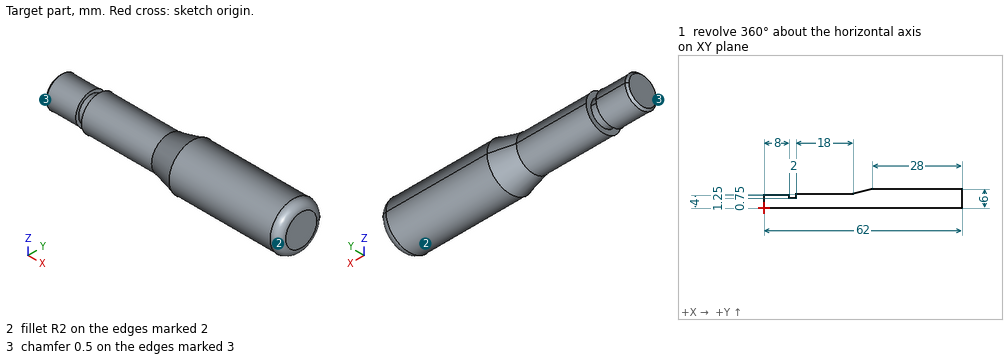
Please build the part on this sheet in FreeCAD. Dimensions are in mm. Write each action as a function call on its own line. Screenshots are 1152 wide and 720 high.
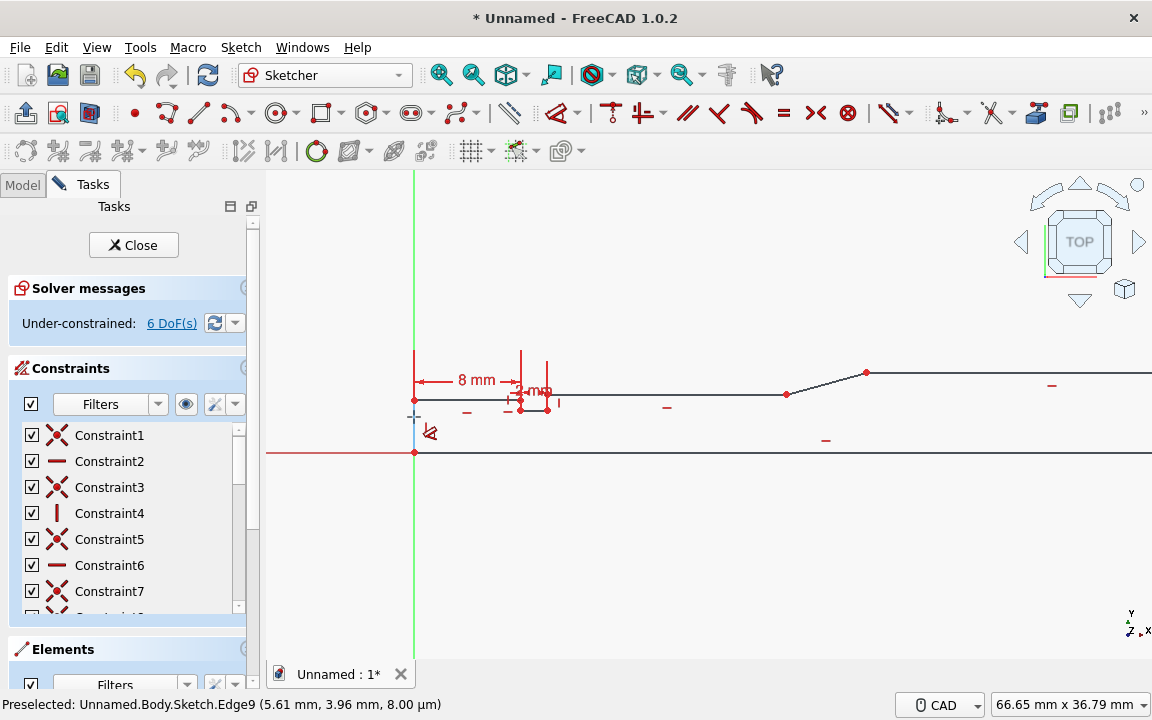
click(414, 416)
click(380, 426)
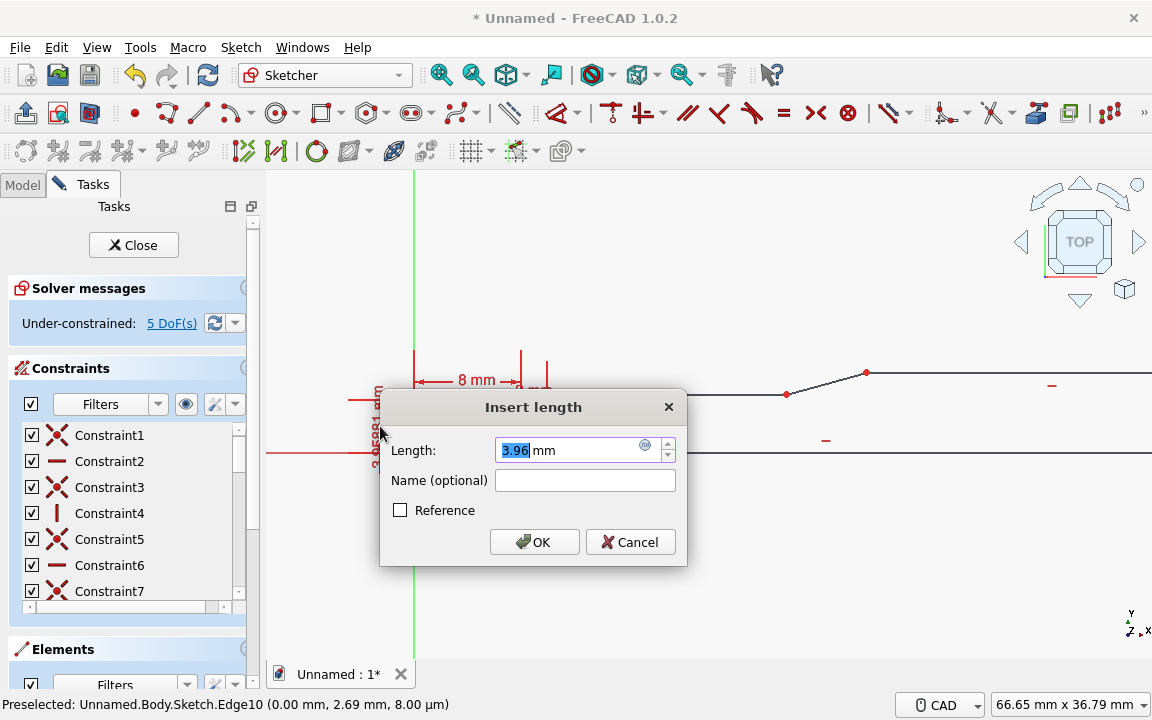
text(4)
key(Return)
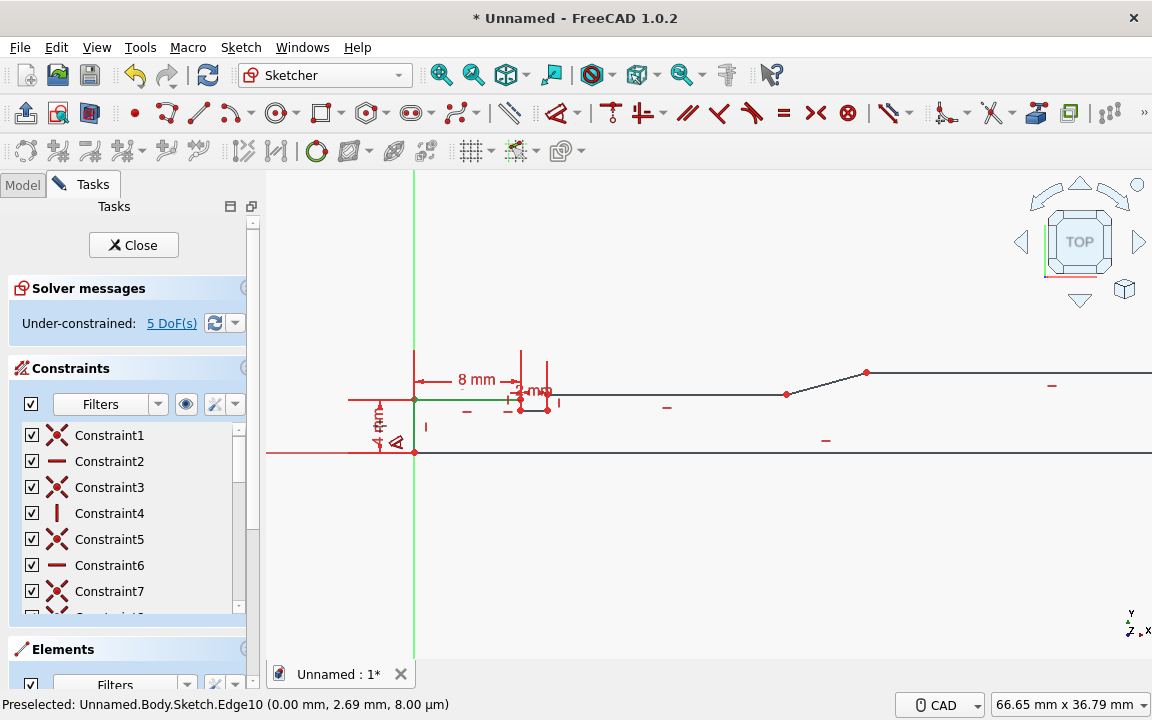
click(662, 453)
click(701, 487)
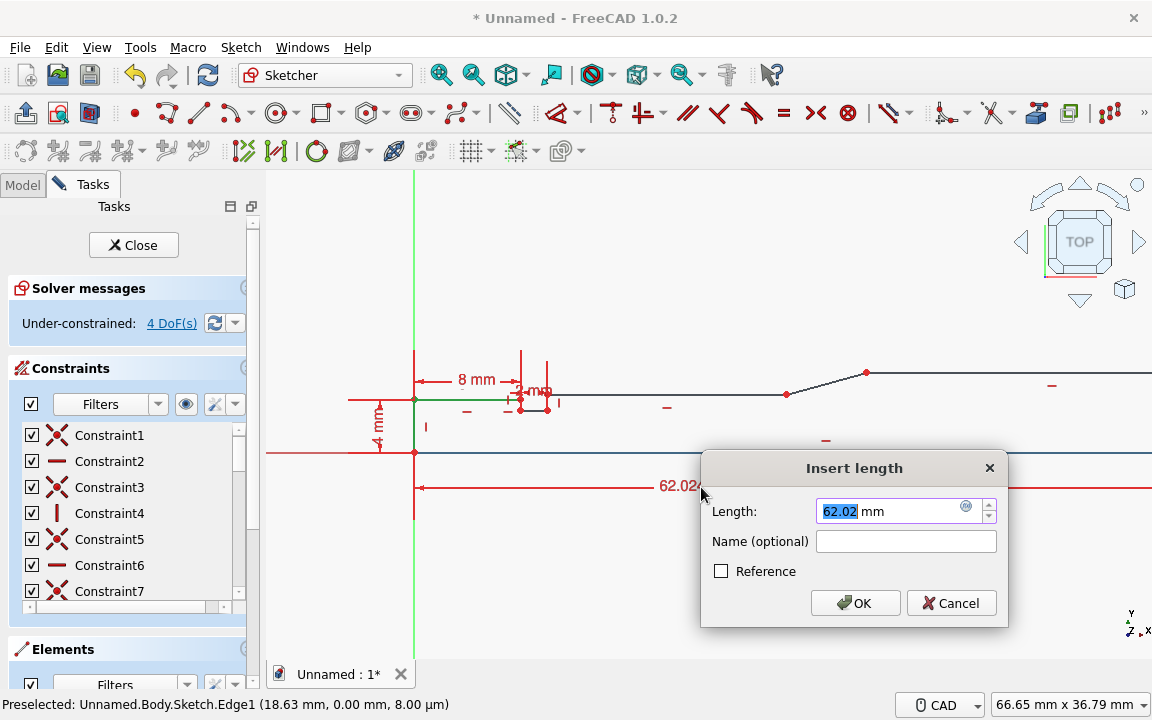
text(62)
key(Return)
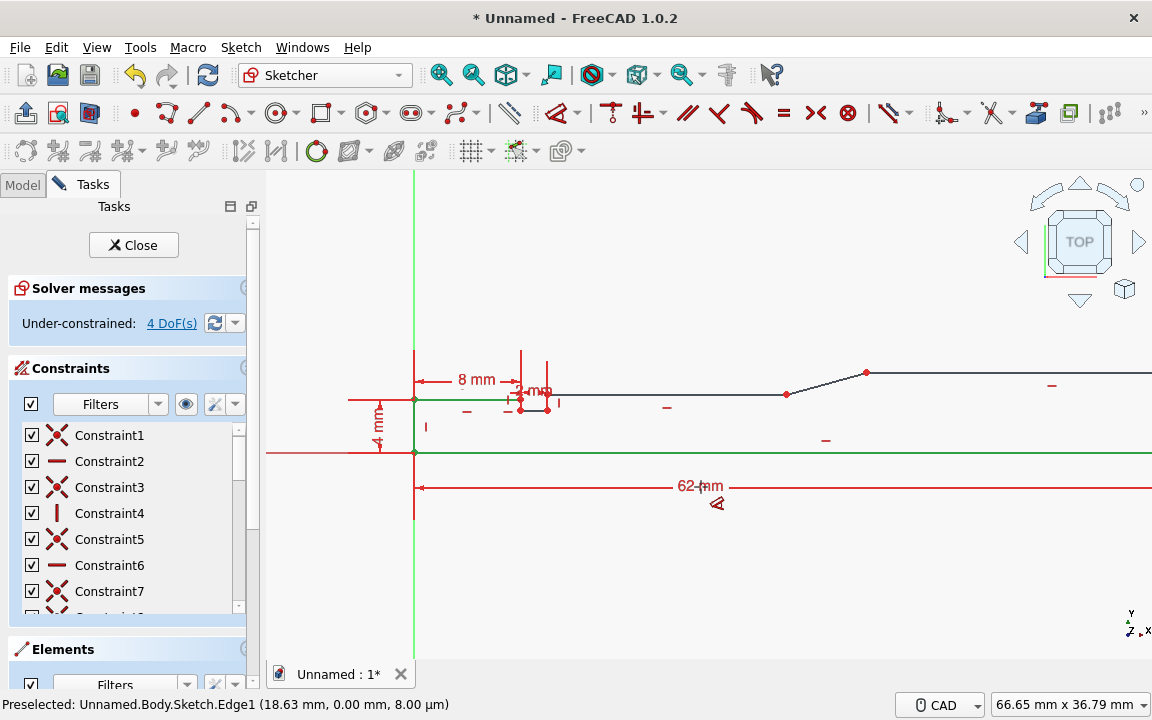
click(978, 373)
click(927, 339)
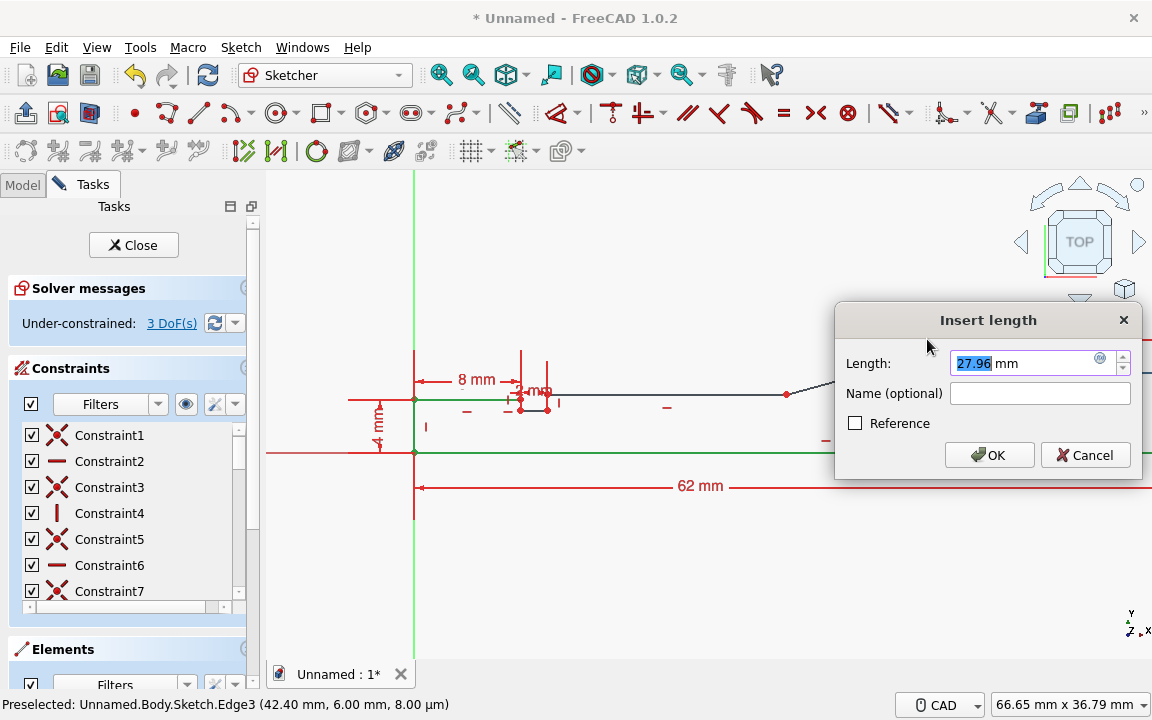
text(28)
key(Return)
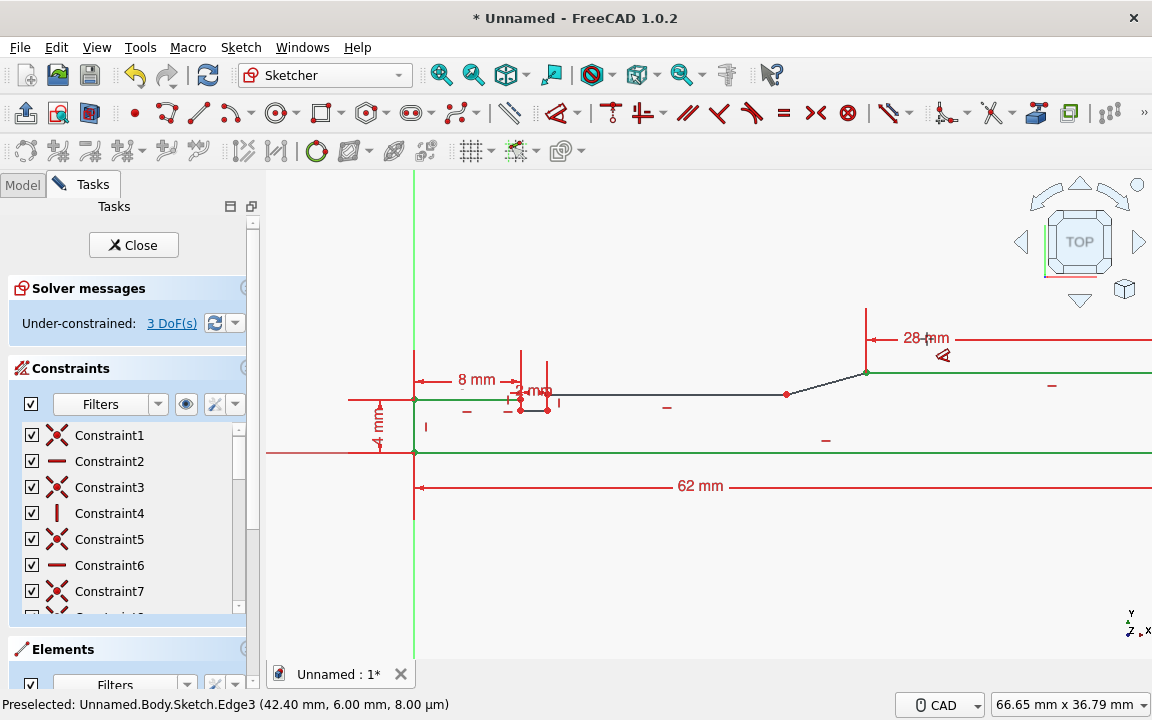
click(715, 395)
click(667, 361)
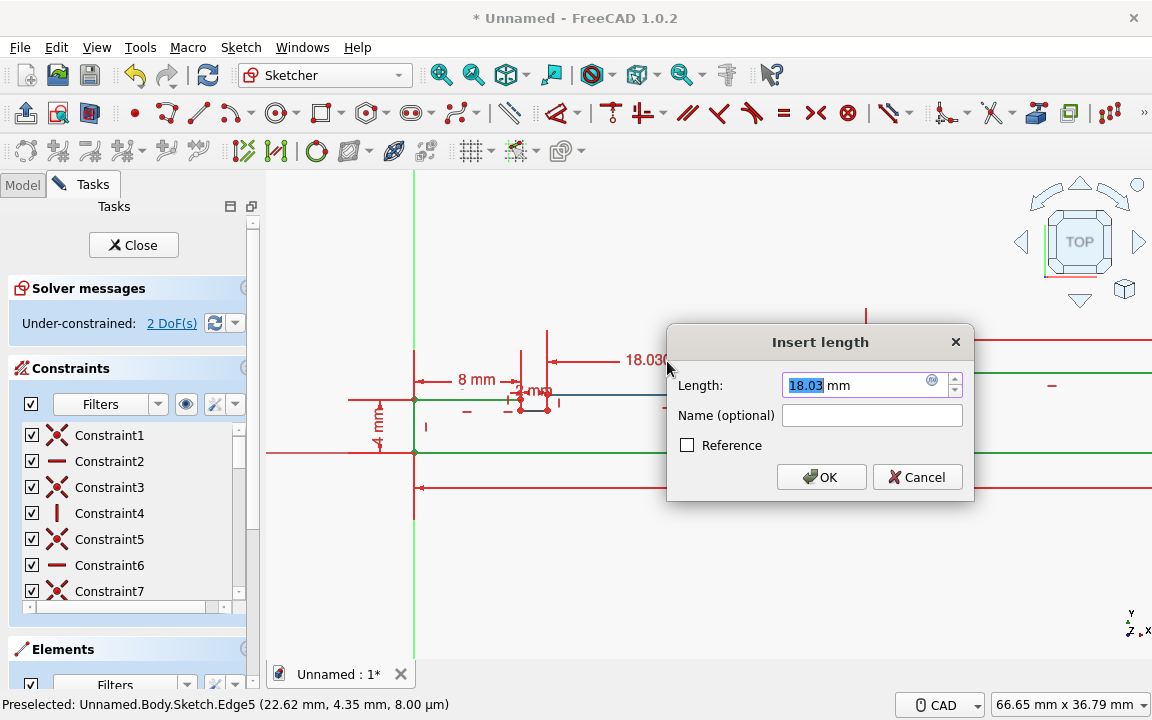
text(18)
key(Return)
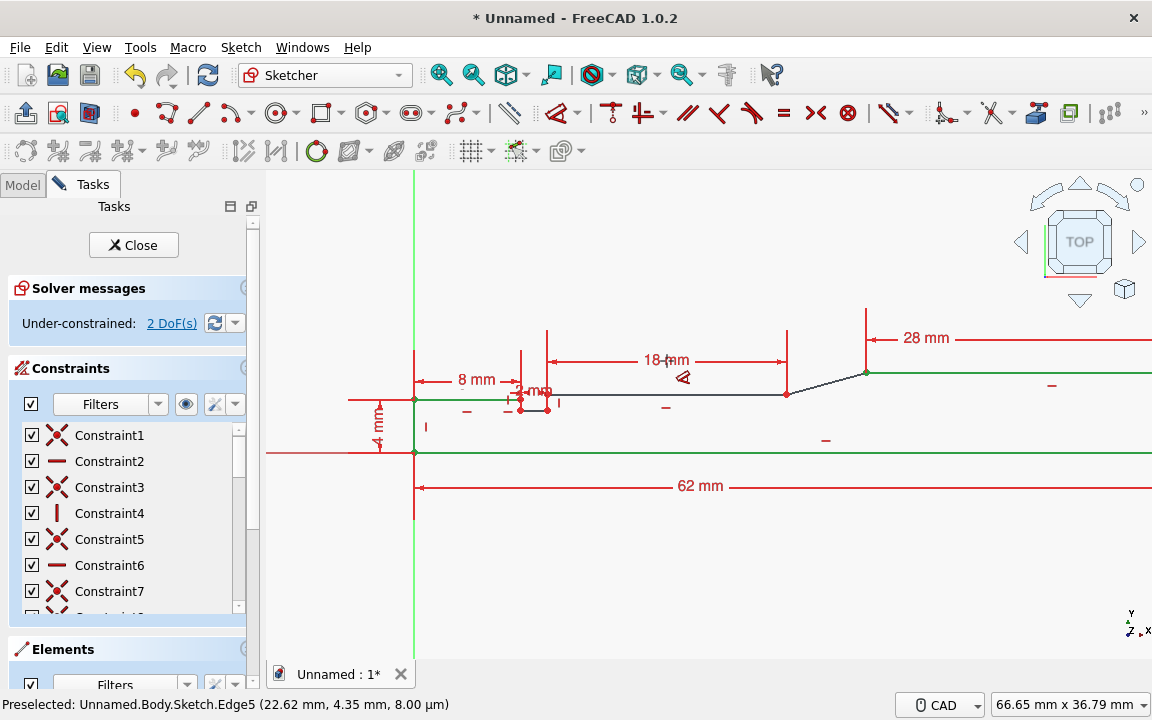
scroll(547, 403, up, 5)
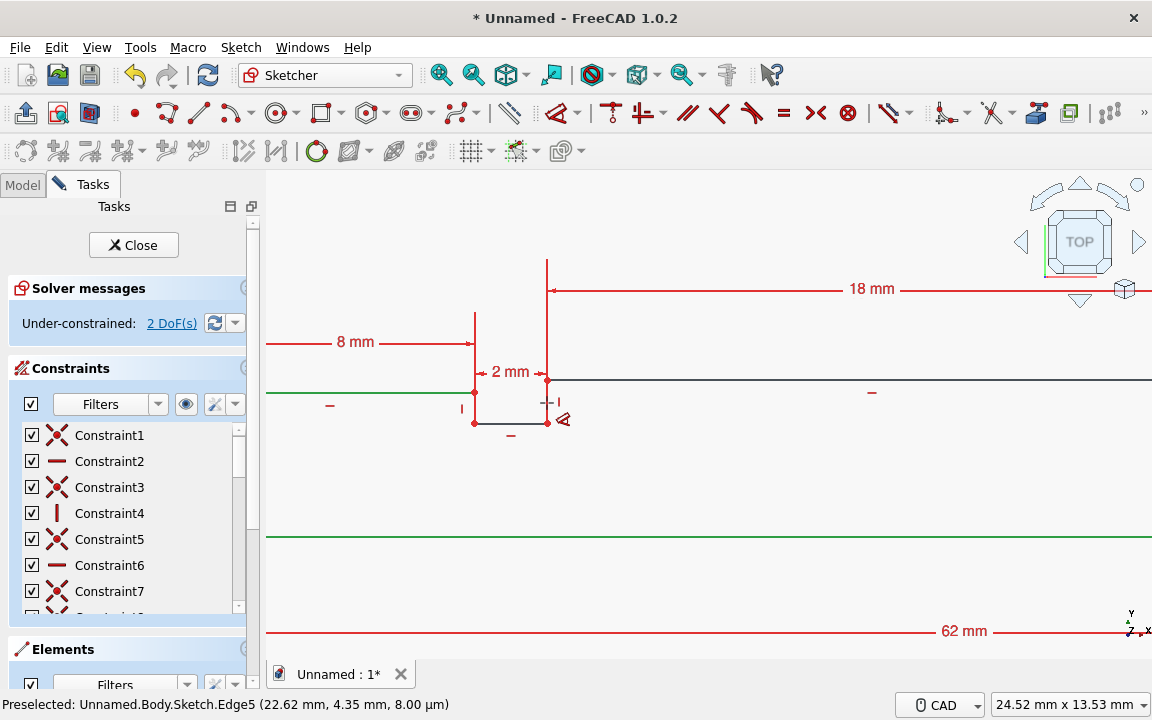
click(547, 402)
click(513, 402)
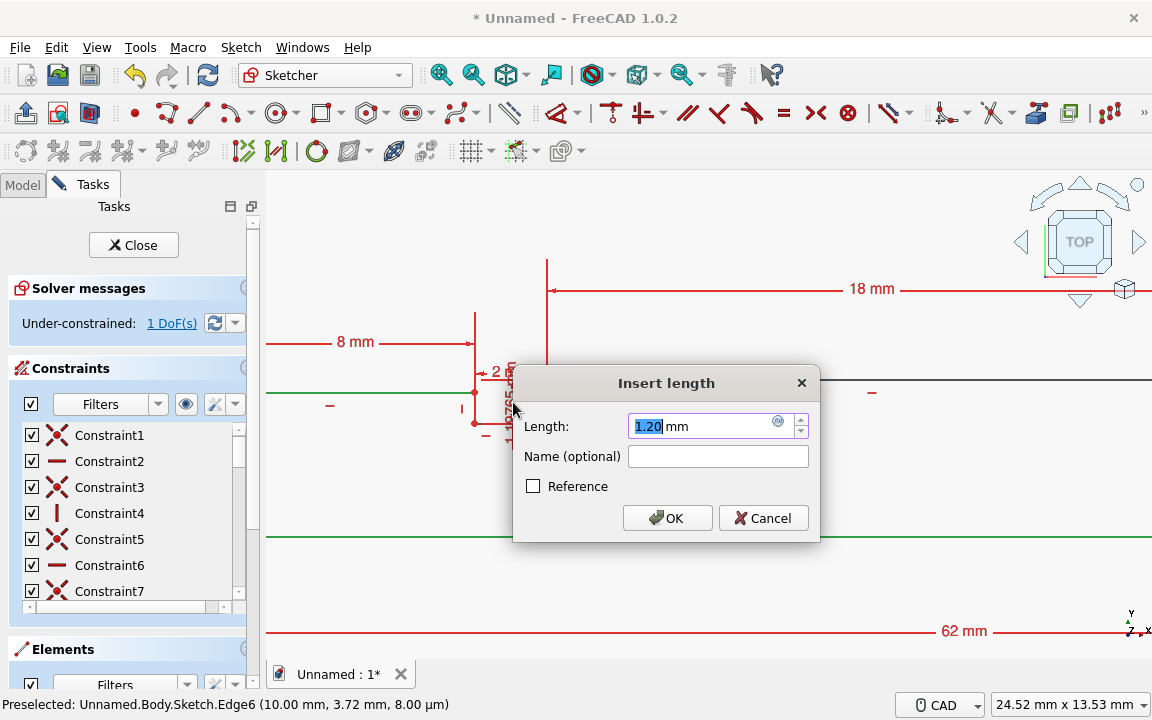
text(1.25)
key(Return)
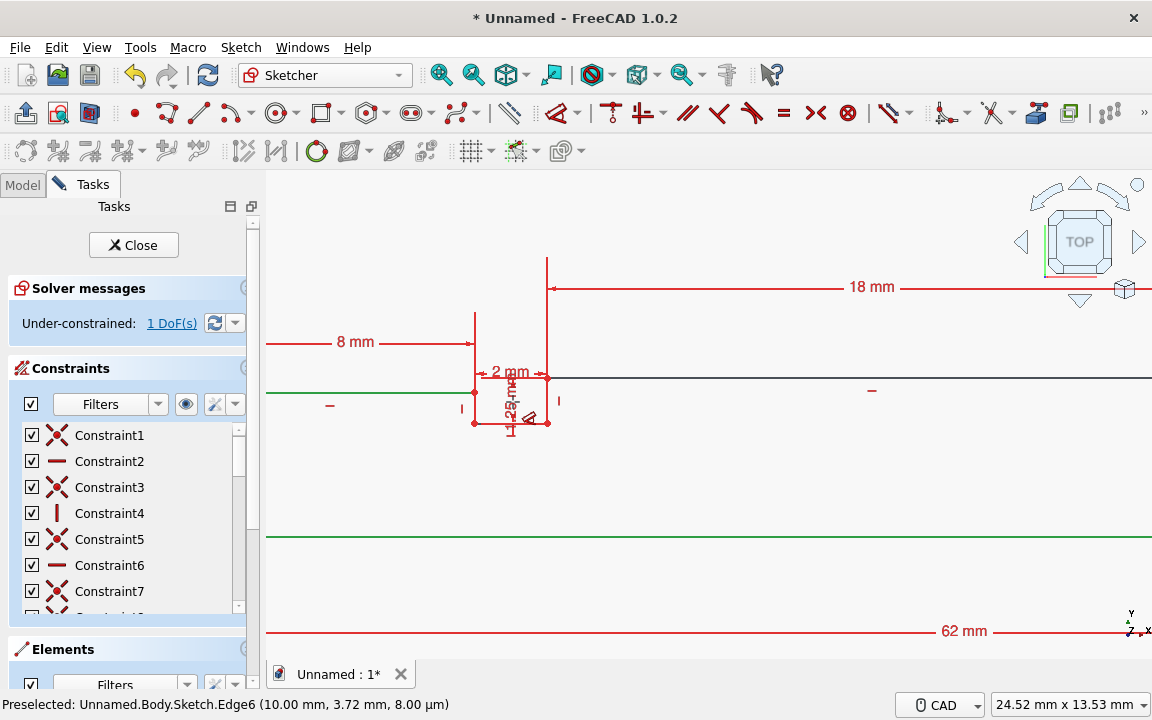
scroll(475, 414, up, 3)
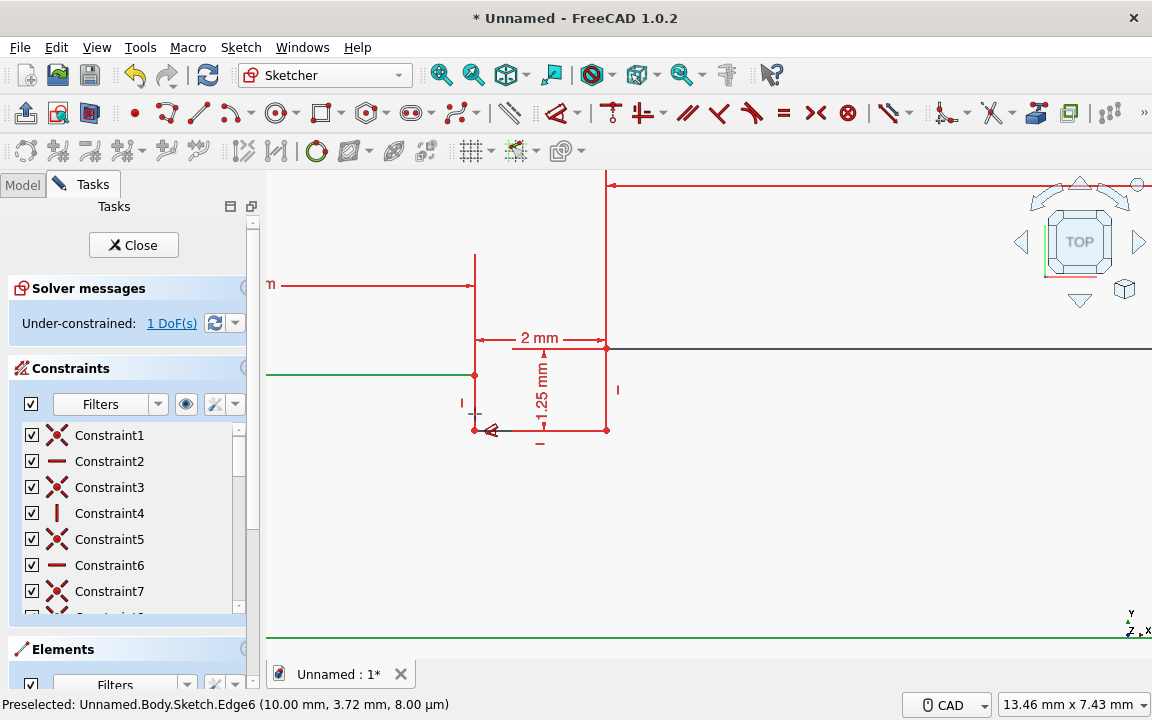
click(475, 414)
click(441, 403)